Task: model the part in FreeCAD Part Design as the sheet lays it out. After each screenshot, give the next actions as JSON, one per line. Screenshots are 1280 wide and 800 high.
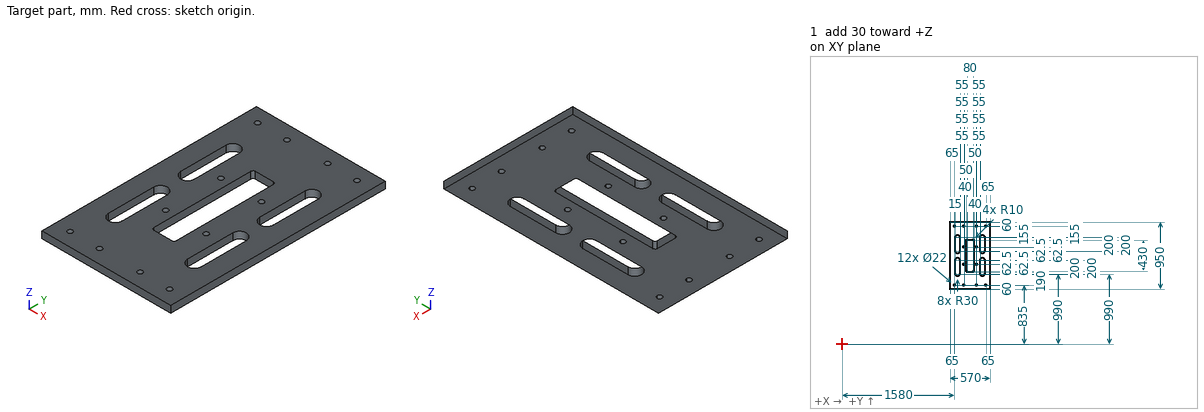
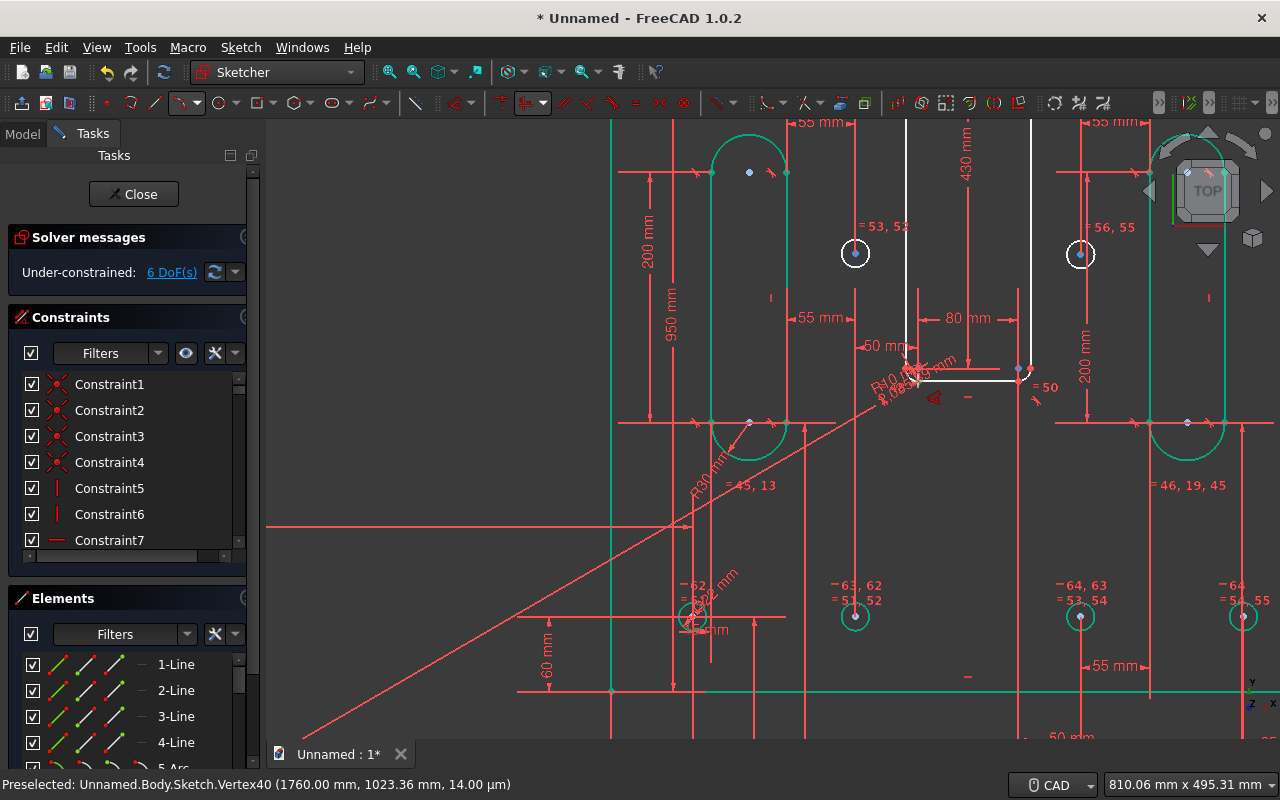
{"action": "scroll", "coordinate": [878, 390], "scroll_direction": "down", "scroll_amount": 8}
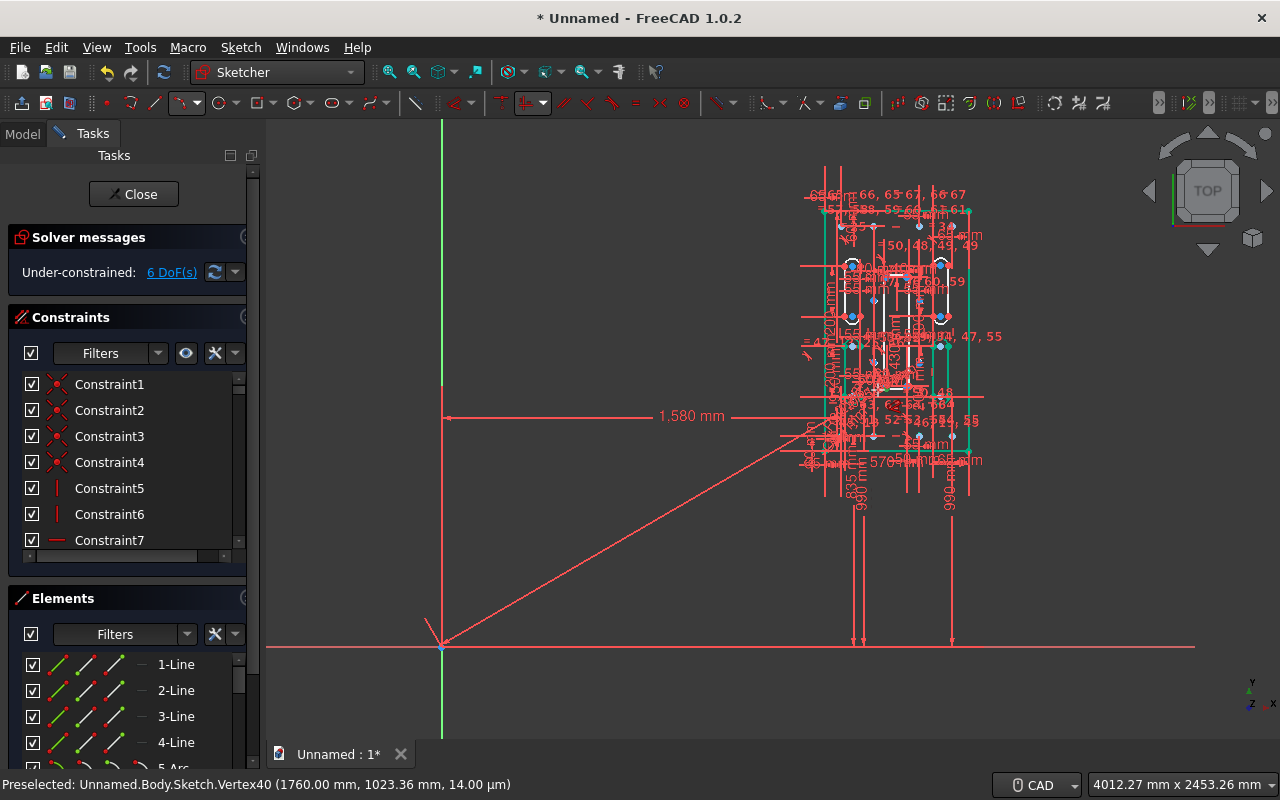
{"action": "left_click", "coordinate": [874, 436]}
{"action": "left_click", "coordinate": [921, 412]}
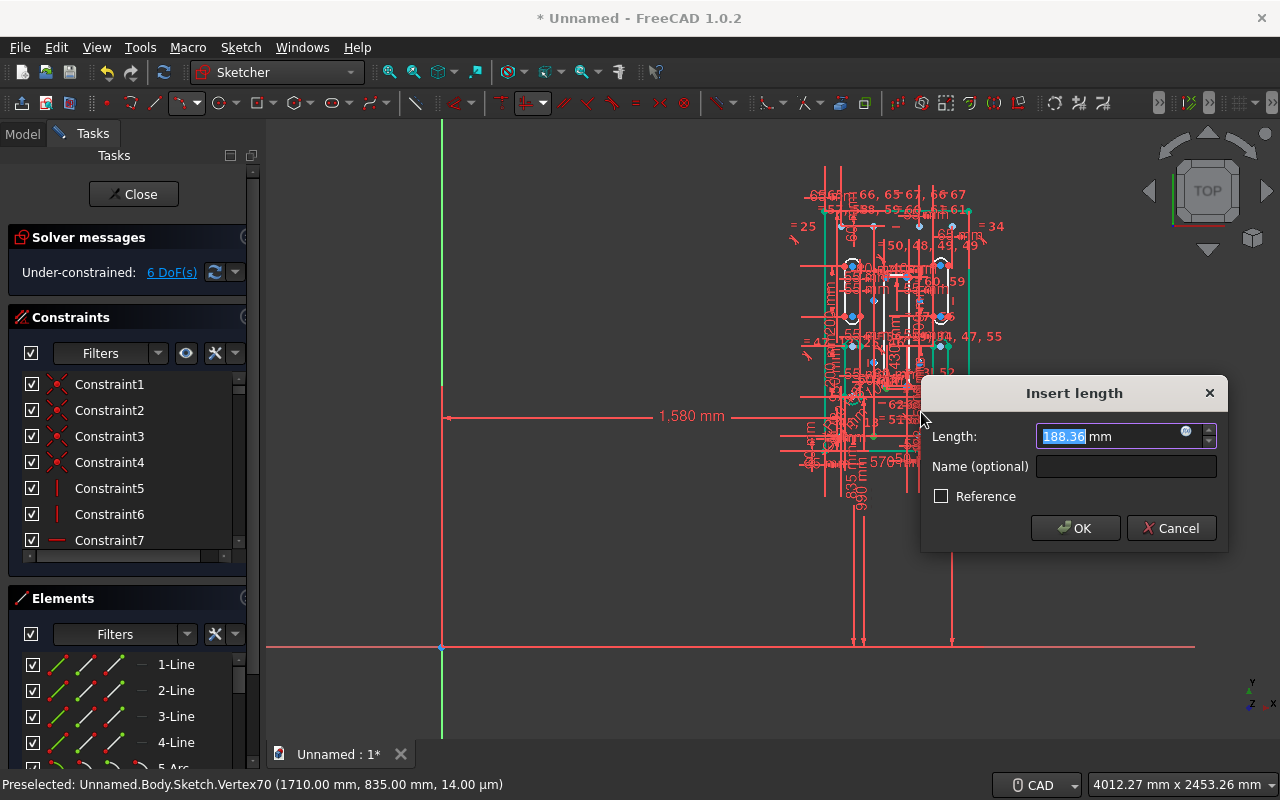
{"action": "type", "text": "190"}
{"action": "key", "text": "Return"}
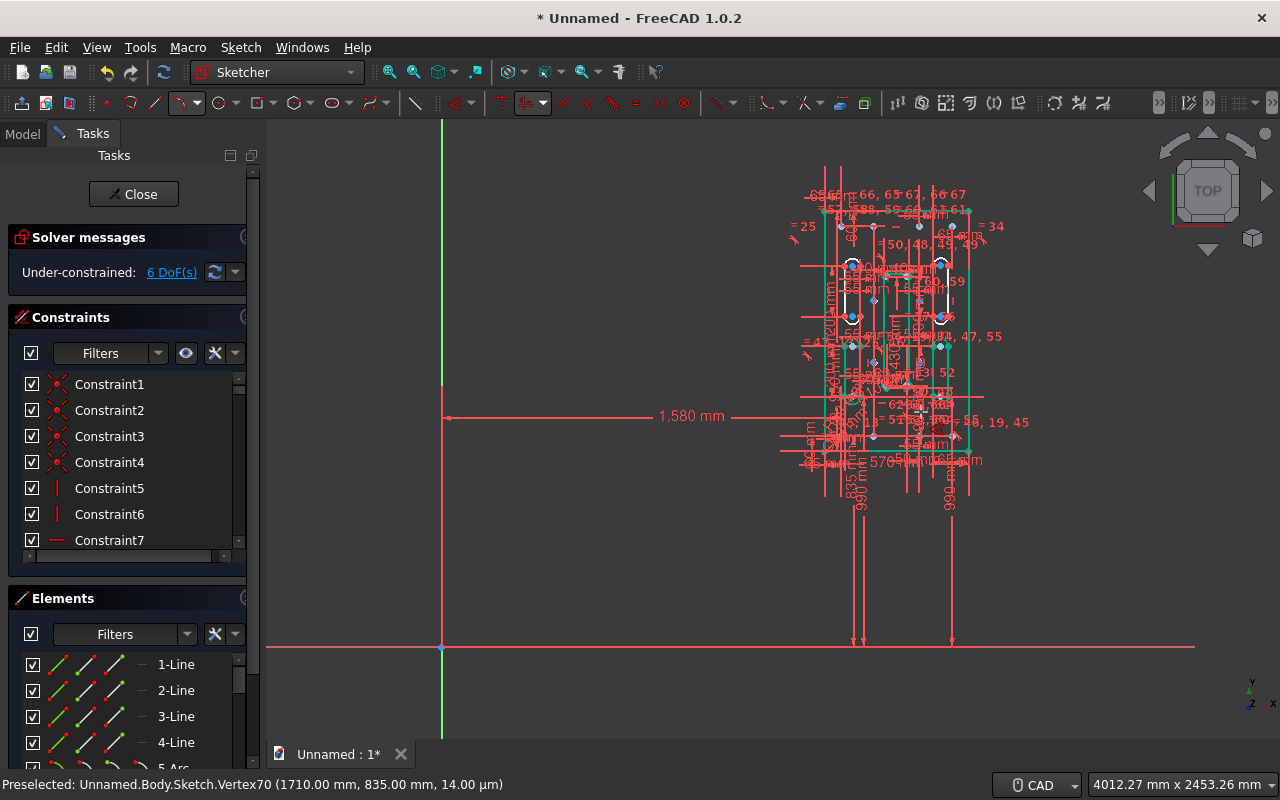
{"action": "scroll", "coordinate": [845, 266], "scroll_direction": "up", "scroll_amount": 3}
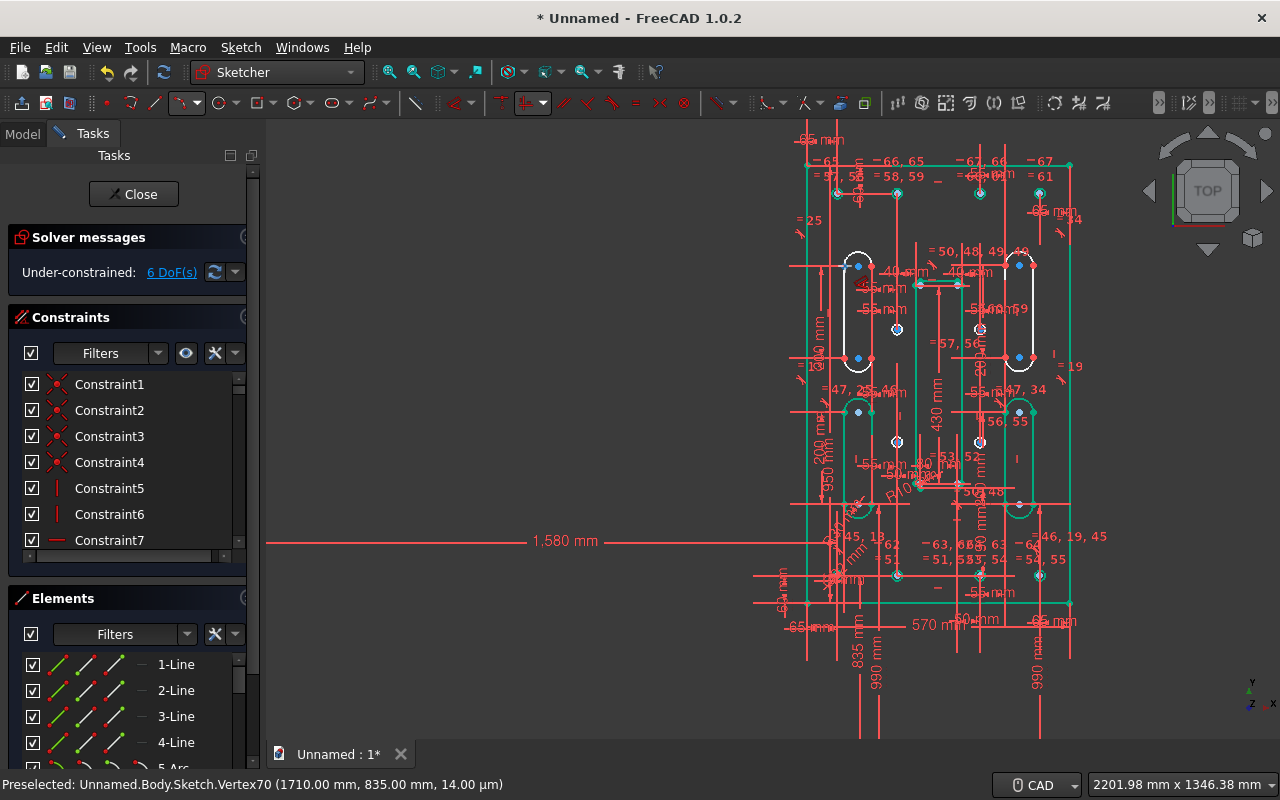
{"action": "left_click", "coordinate": [844, 266]}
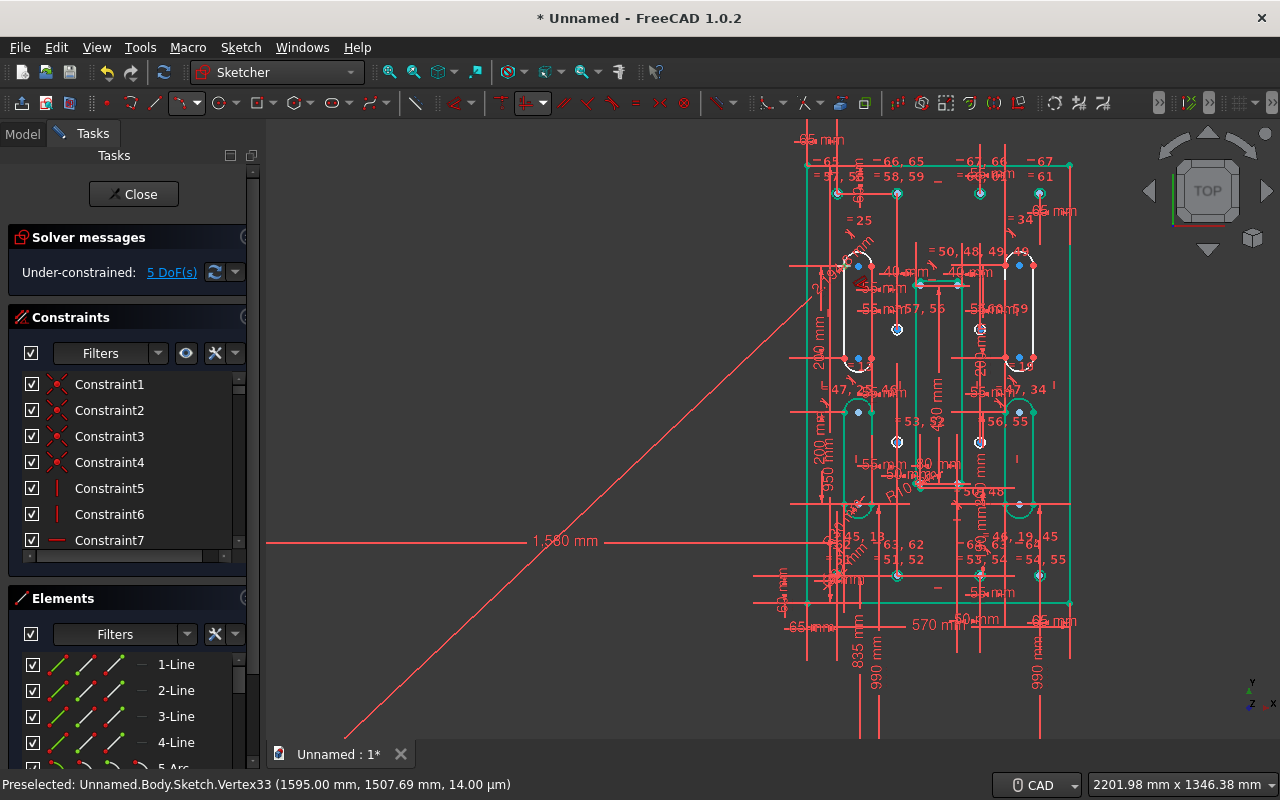
{"action": "left_click", "coordinate": [837, 194]}
{"action": "left_click", "coordinate": [878, 230]}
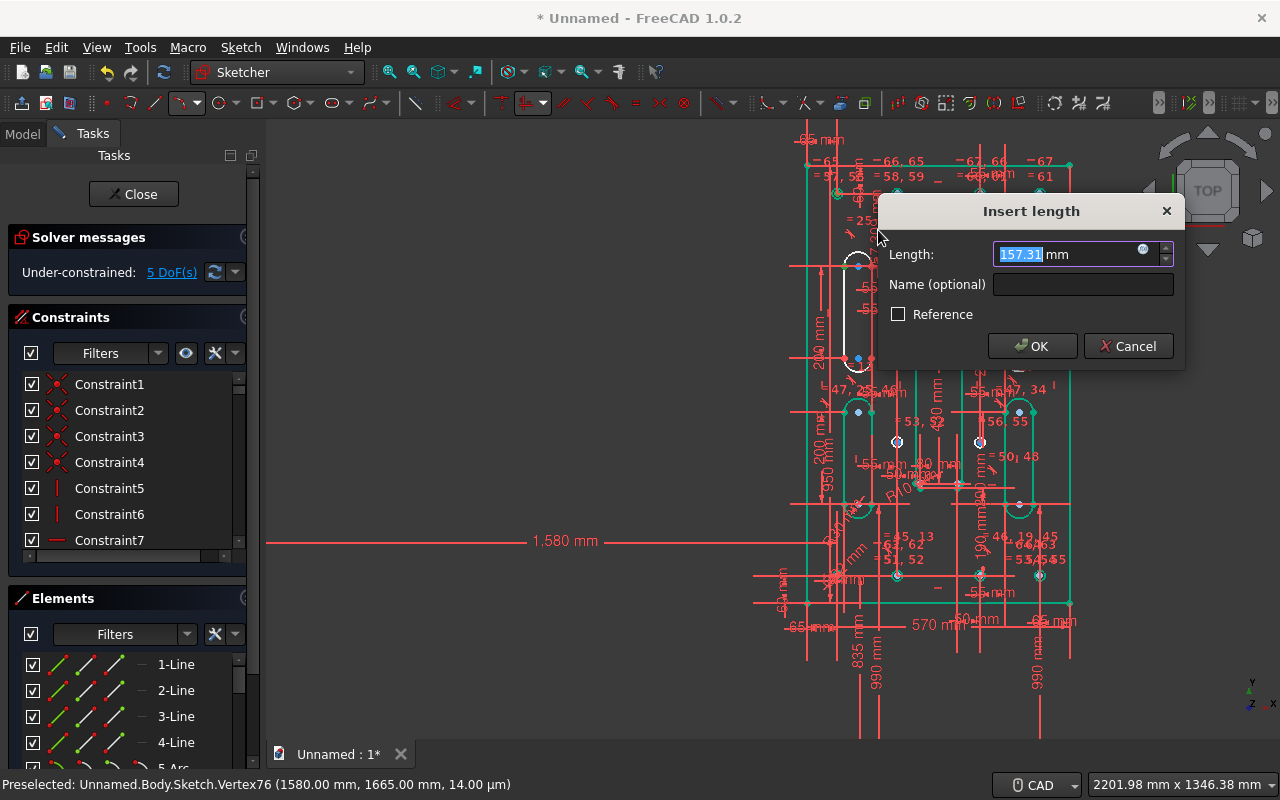
{"action": "type", "text": "155"}
{"action": "key", "text": "Return"}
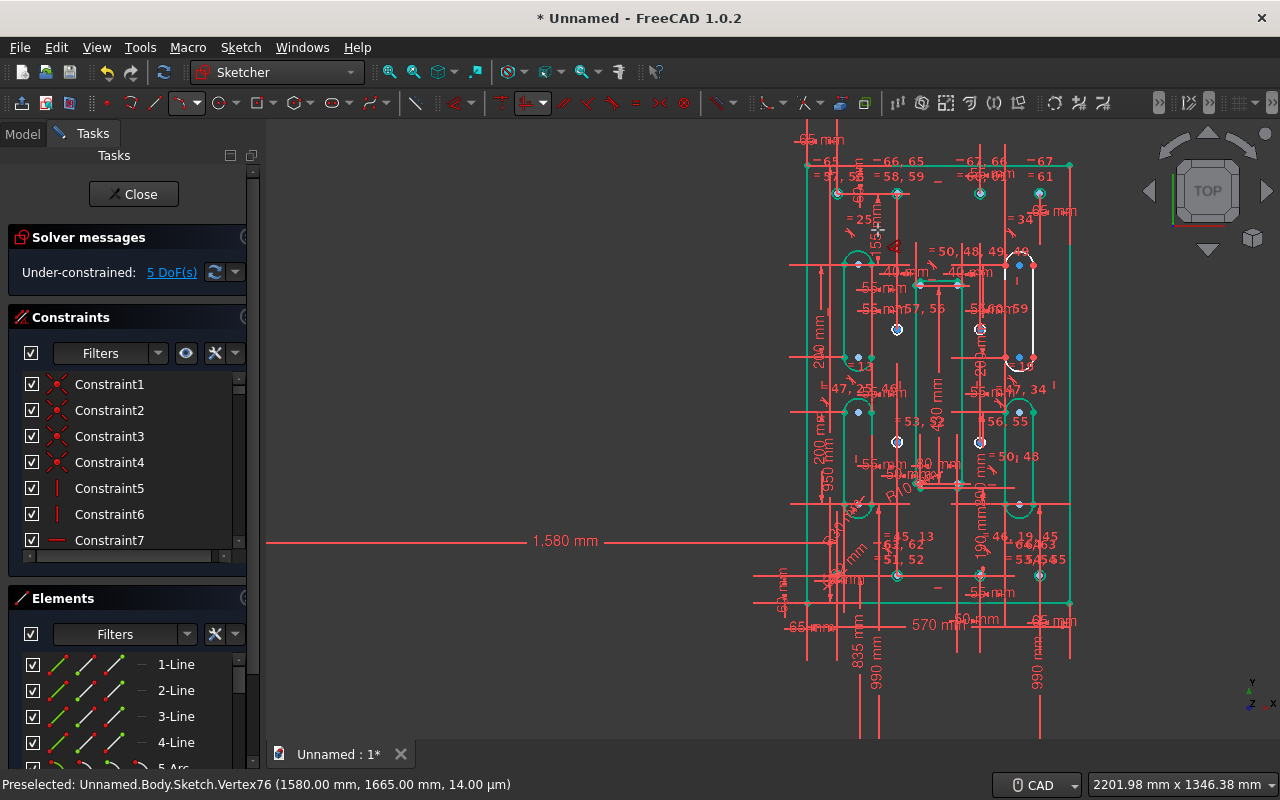
{"action": "left_click", "coordinate": [1005, 265]}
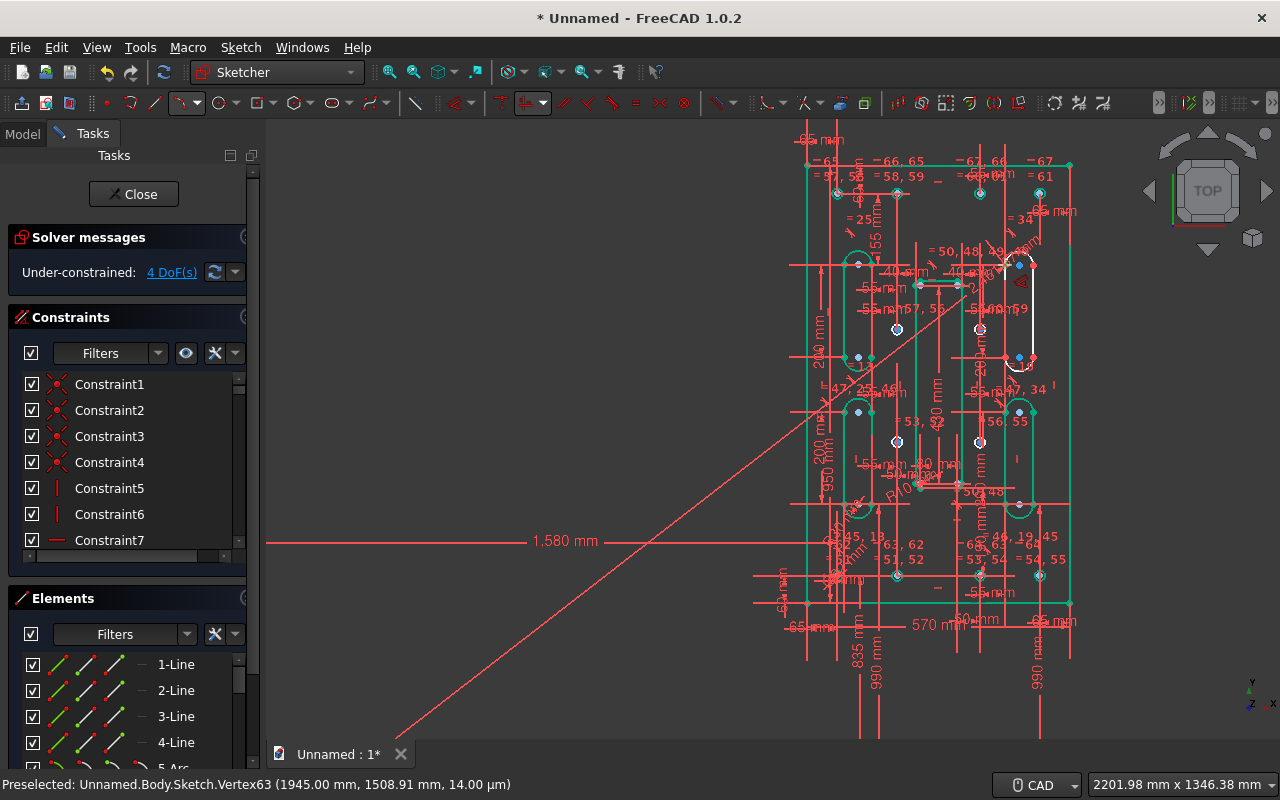
{"action": "left_click", "coordinate": [980, 194]}
{"action": "left_click", "coordinate": [1039, 246]}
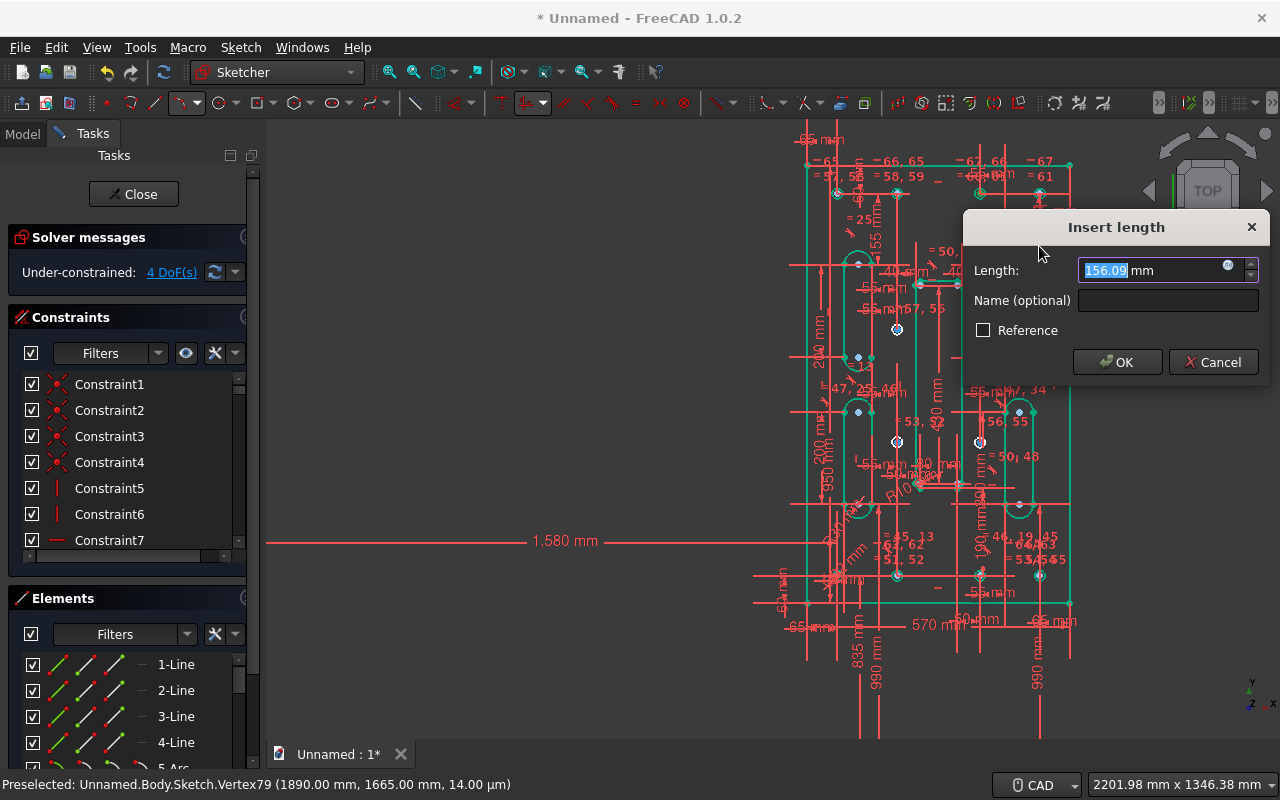
{"action": "type", "text": "155"}
{"action": "key", "text": "Return"}